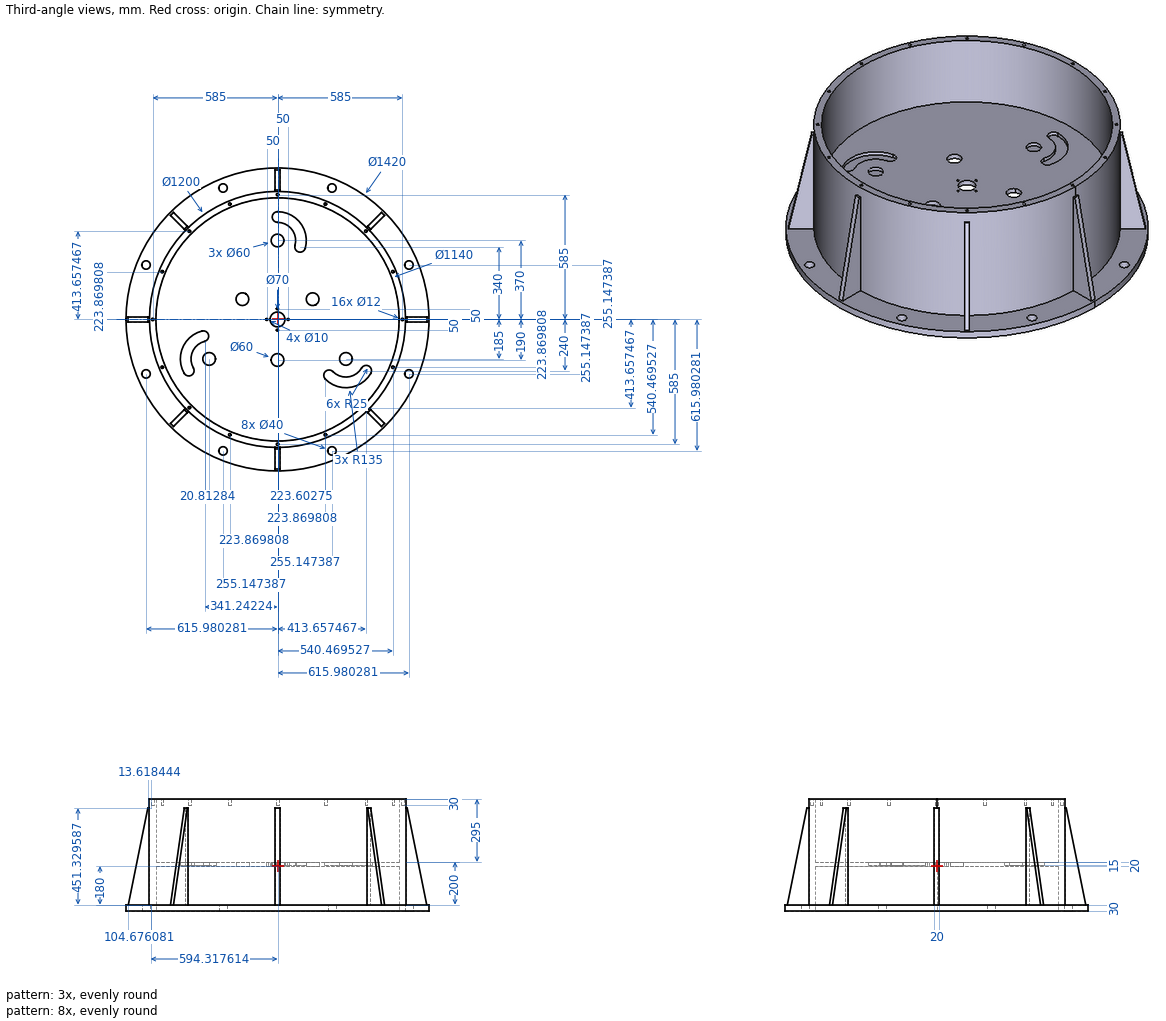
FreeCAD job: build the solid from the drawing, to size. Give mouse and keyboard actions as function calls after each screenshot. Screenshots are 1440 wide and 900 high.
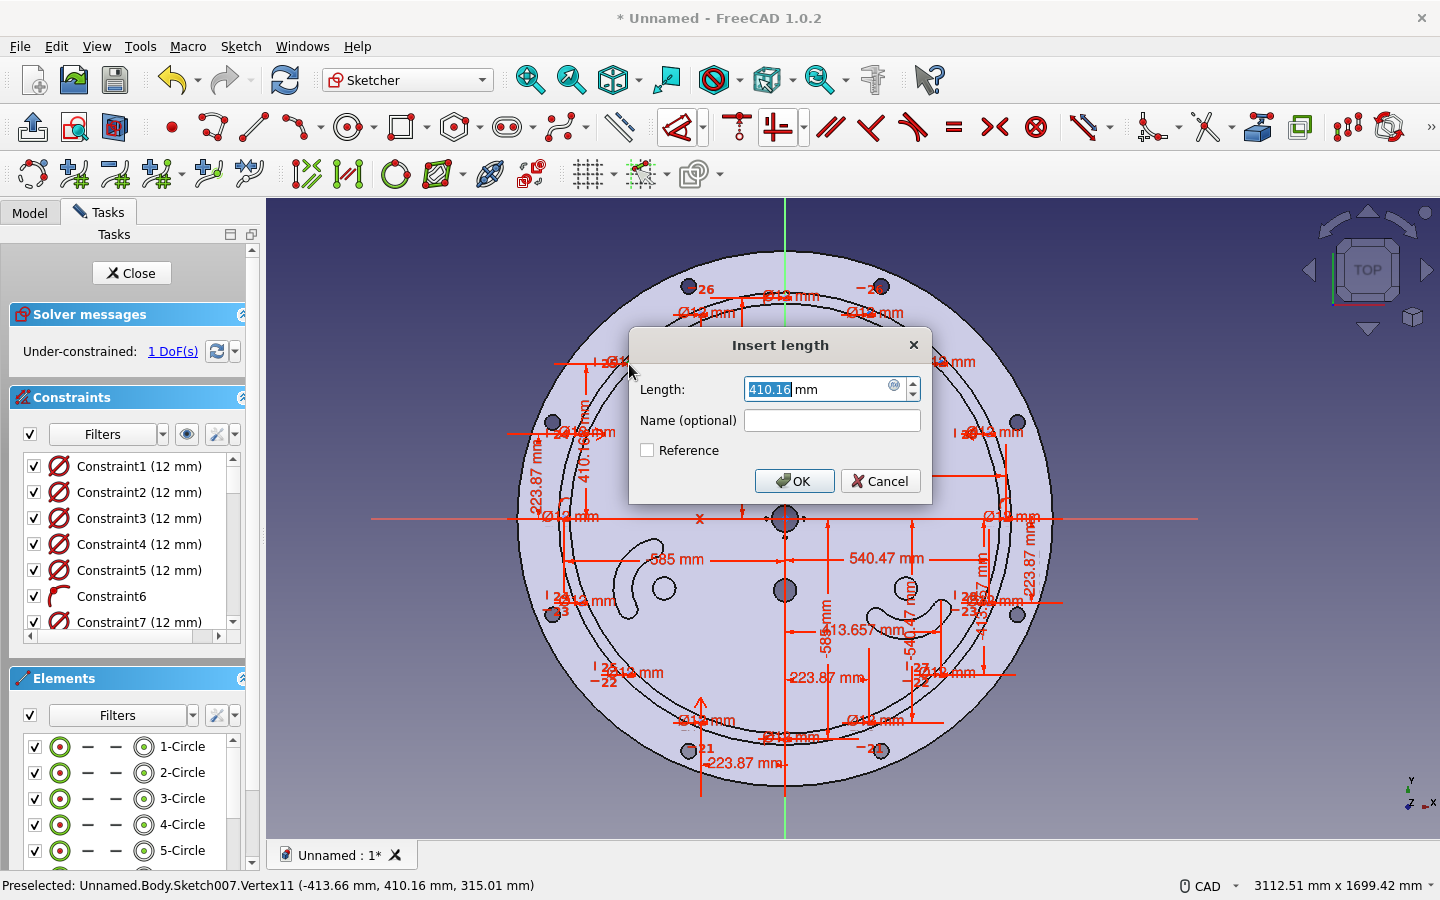
text(413.657467)
key(Return)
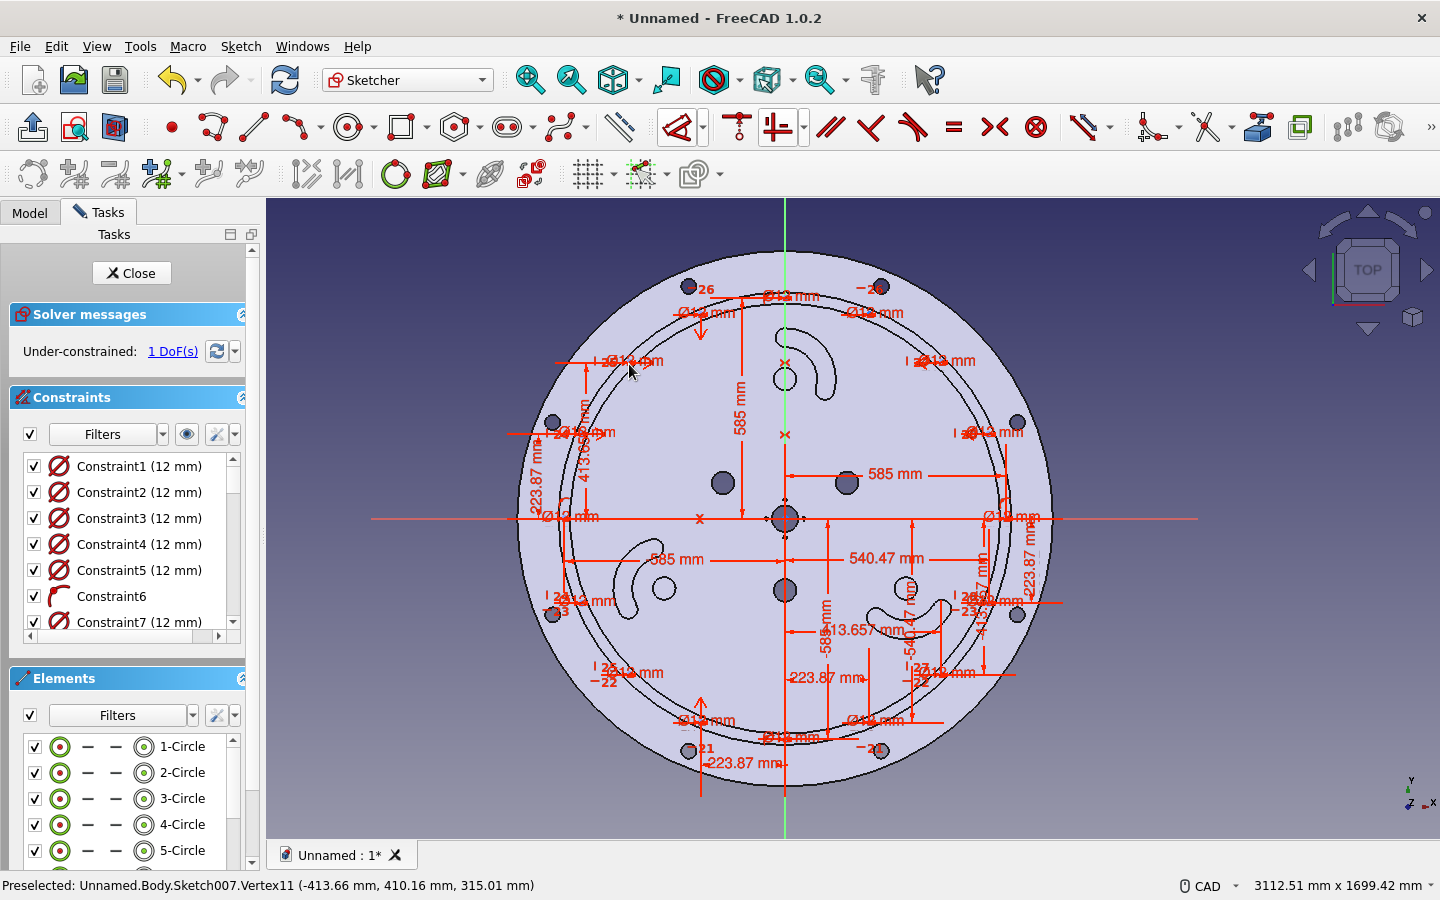
click(869, 315)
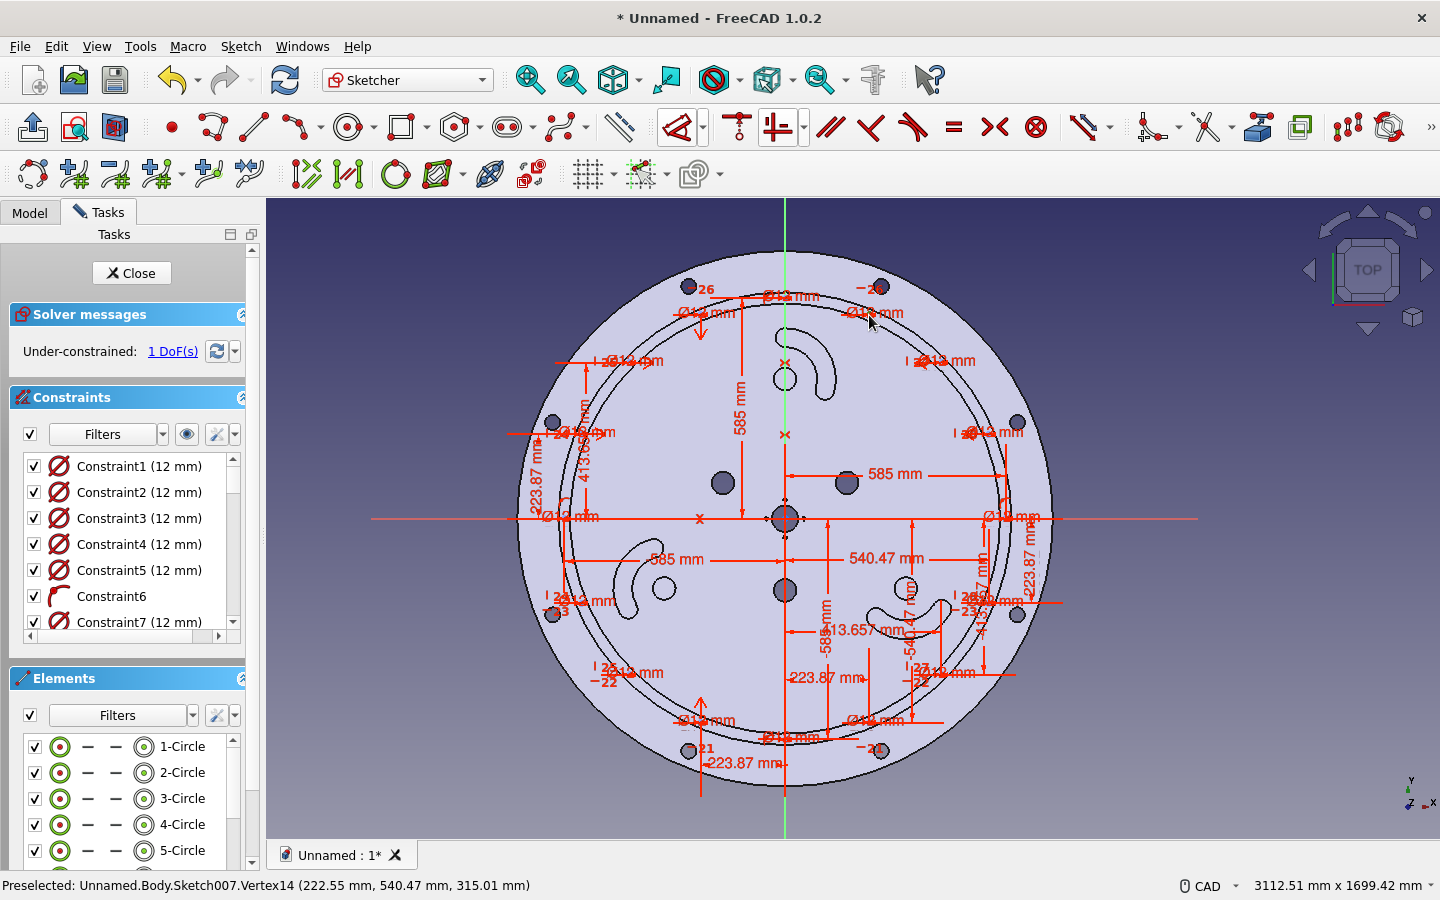
key(l)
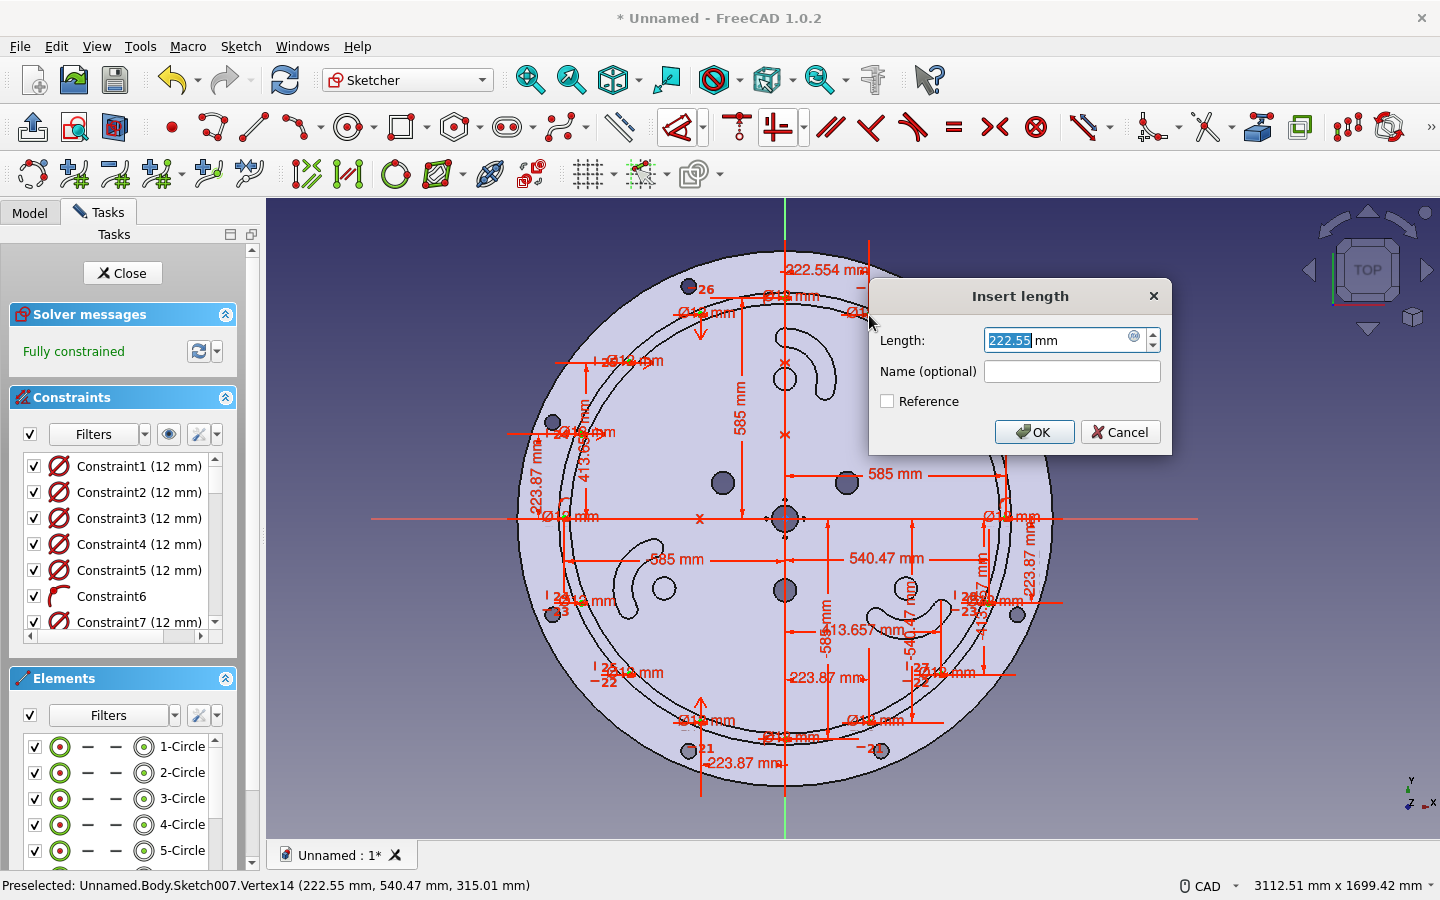
text(223.869808)
key(Return)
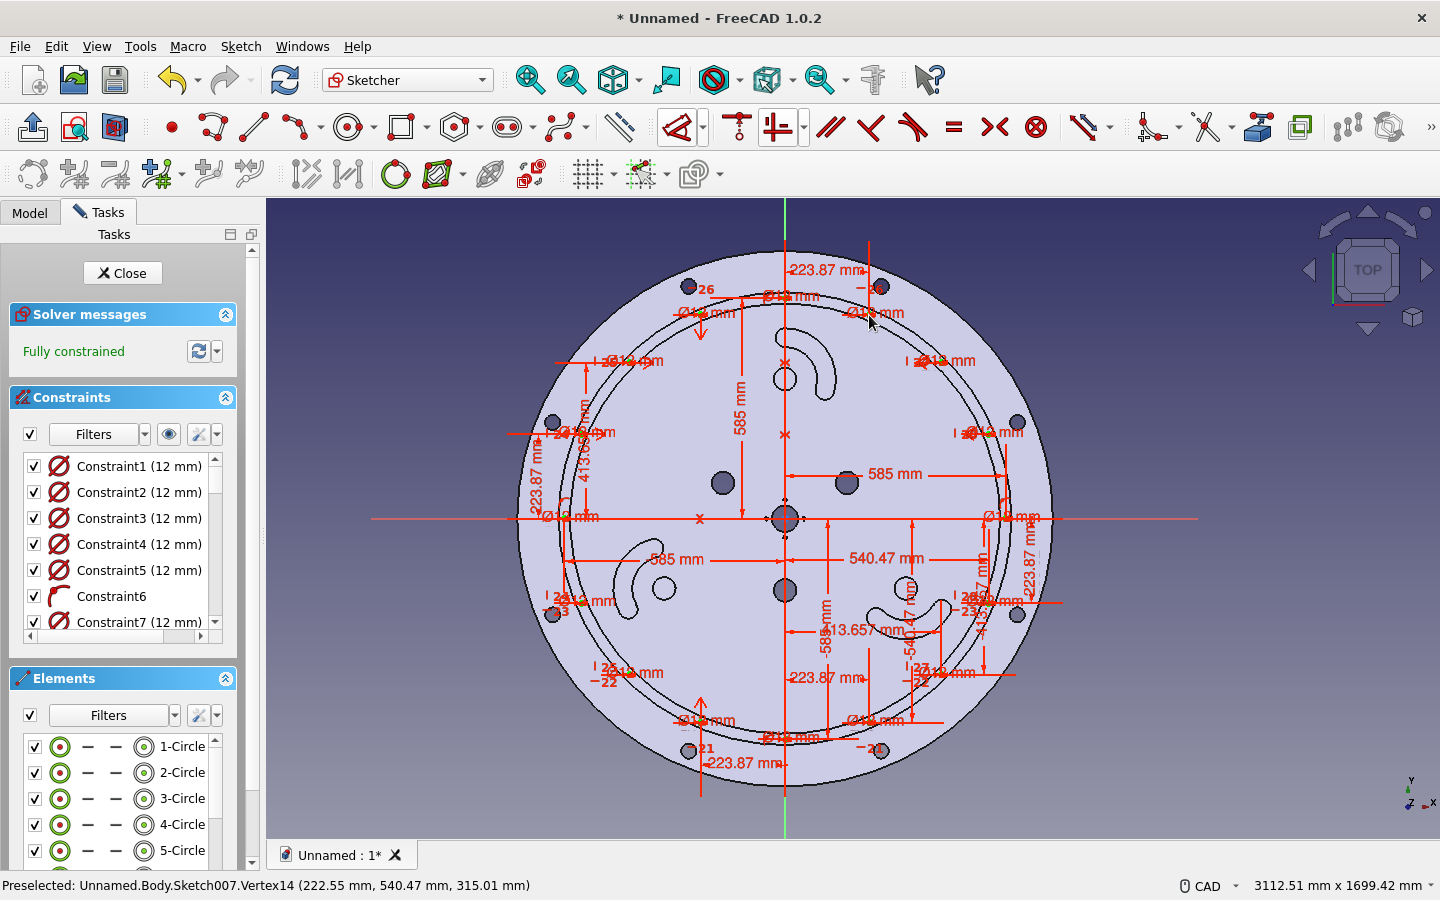
click(123, 273)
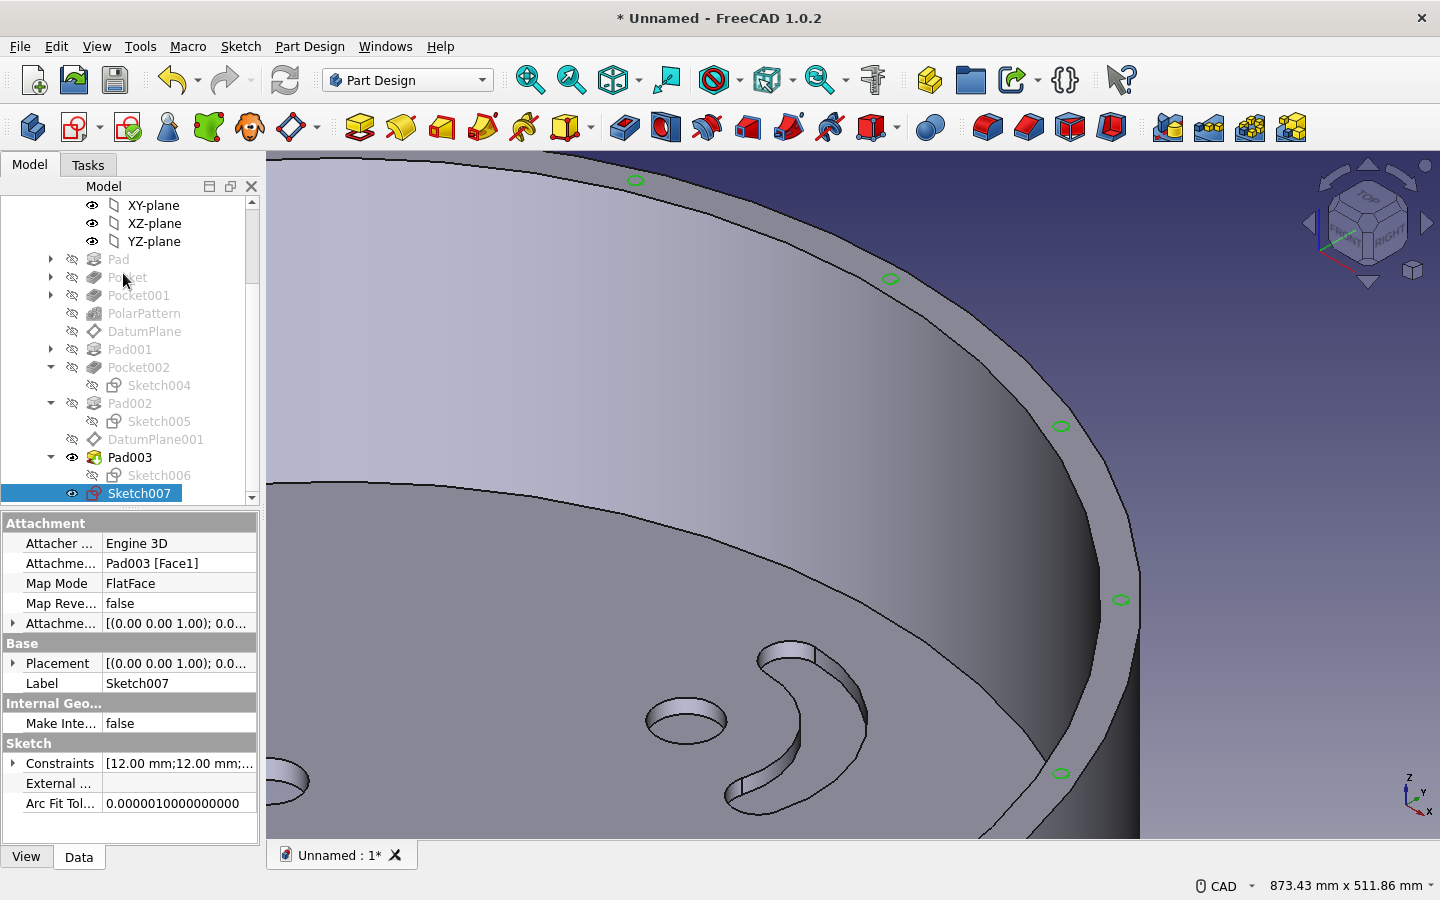
click(625, 128)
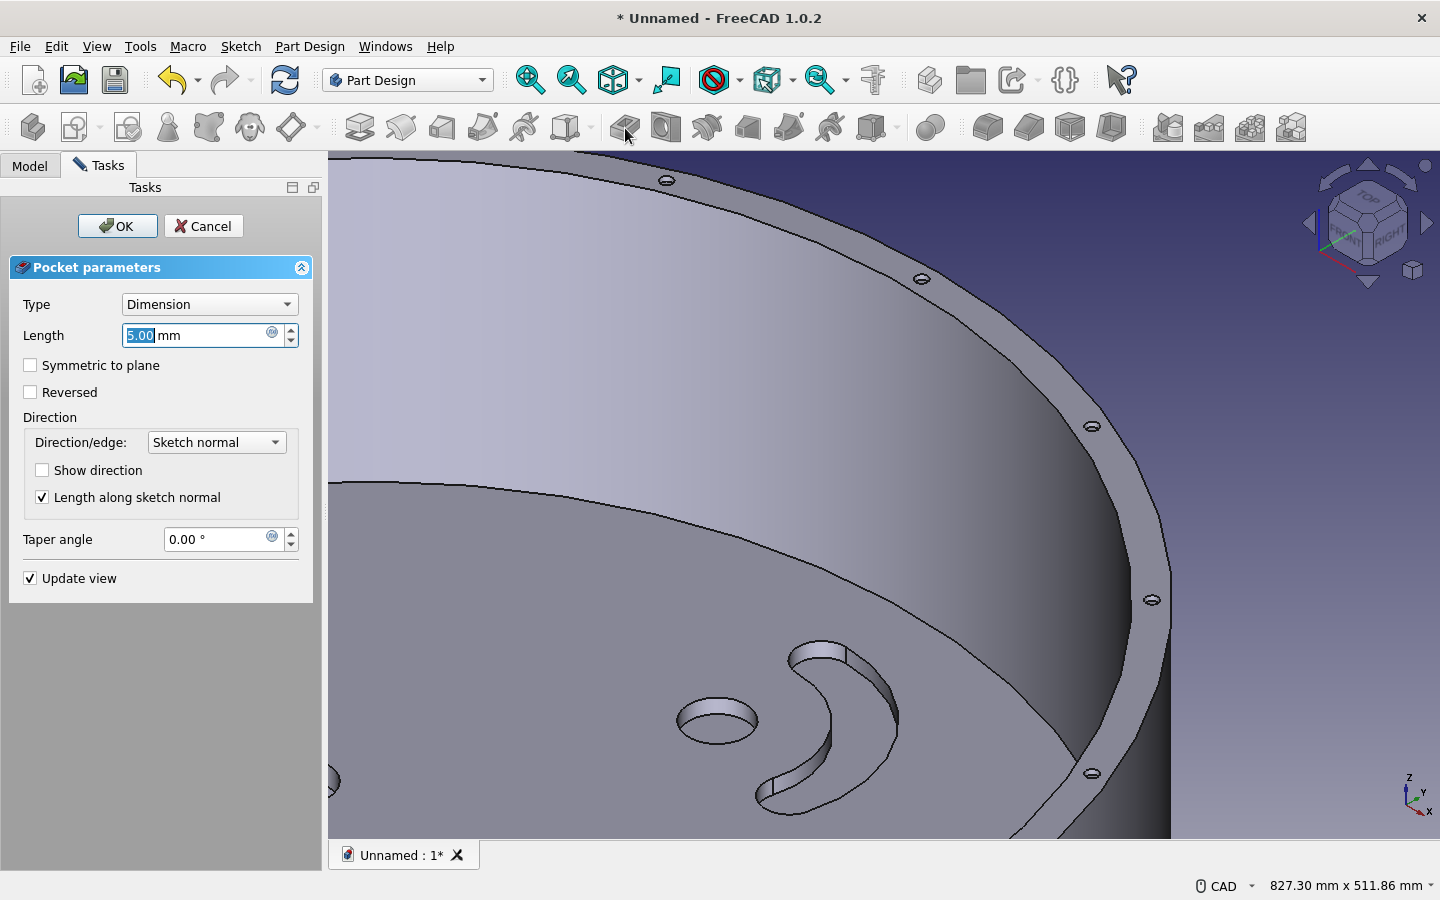
text(30)
key(Tab)